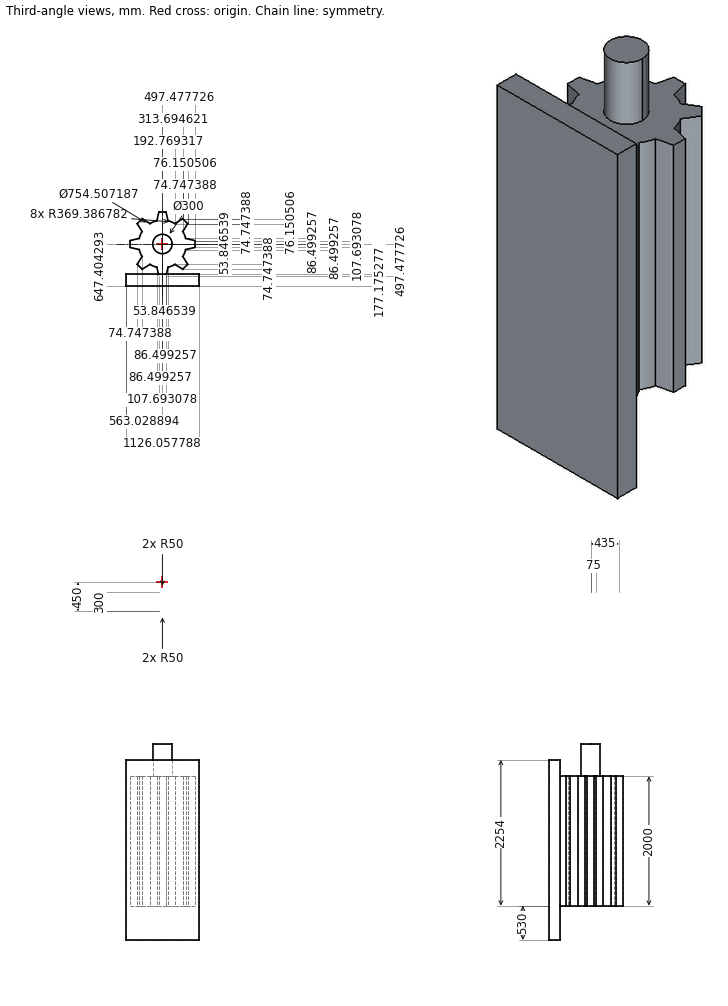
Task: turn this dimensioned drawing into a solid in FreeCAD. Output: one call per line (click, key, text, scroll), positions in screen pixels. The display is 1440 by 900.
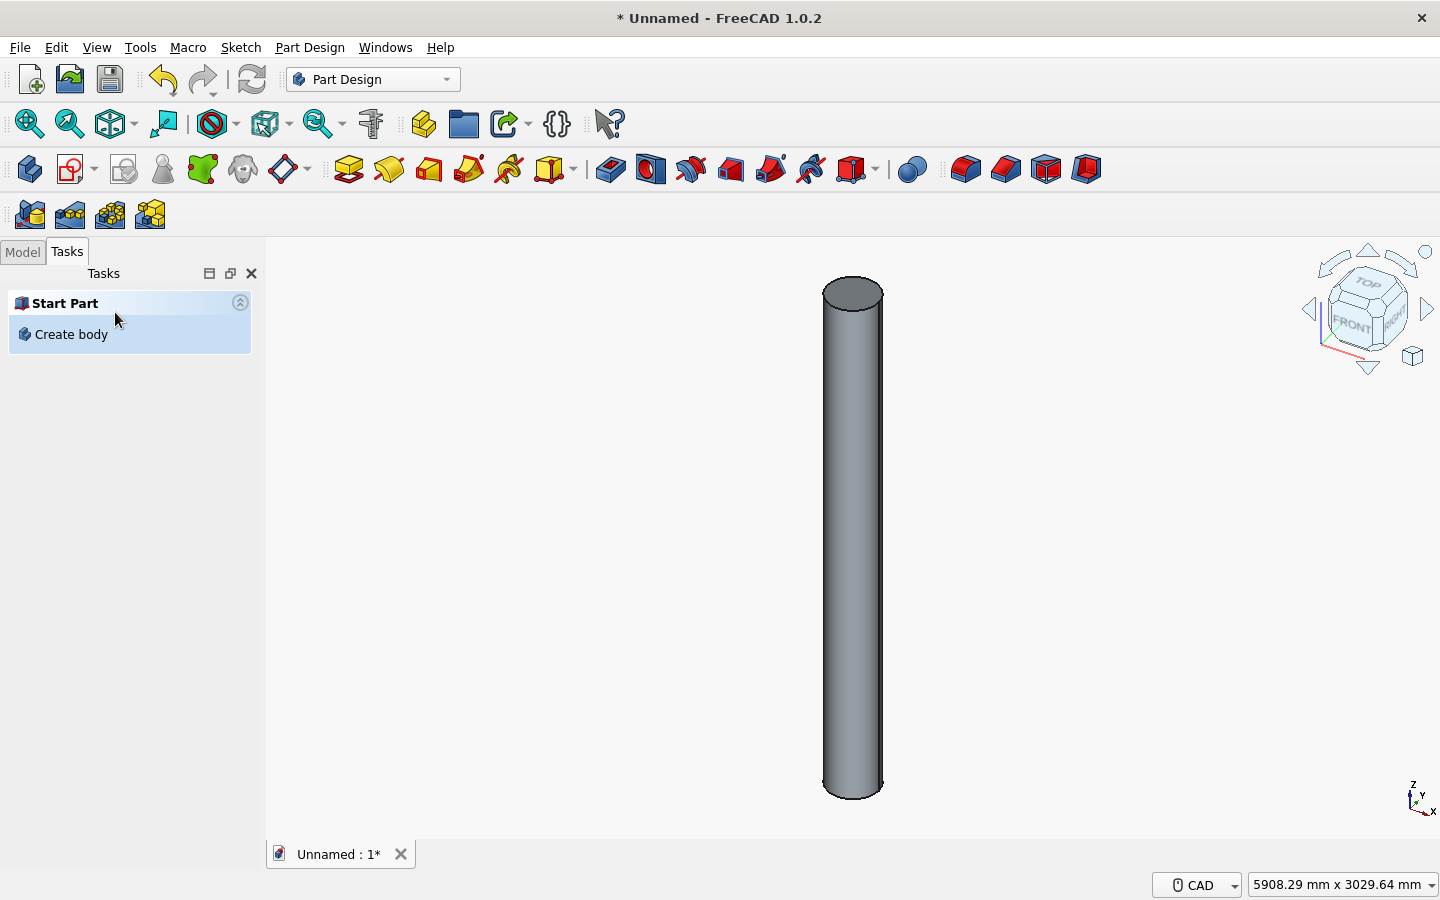
key(5)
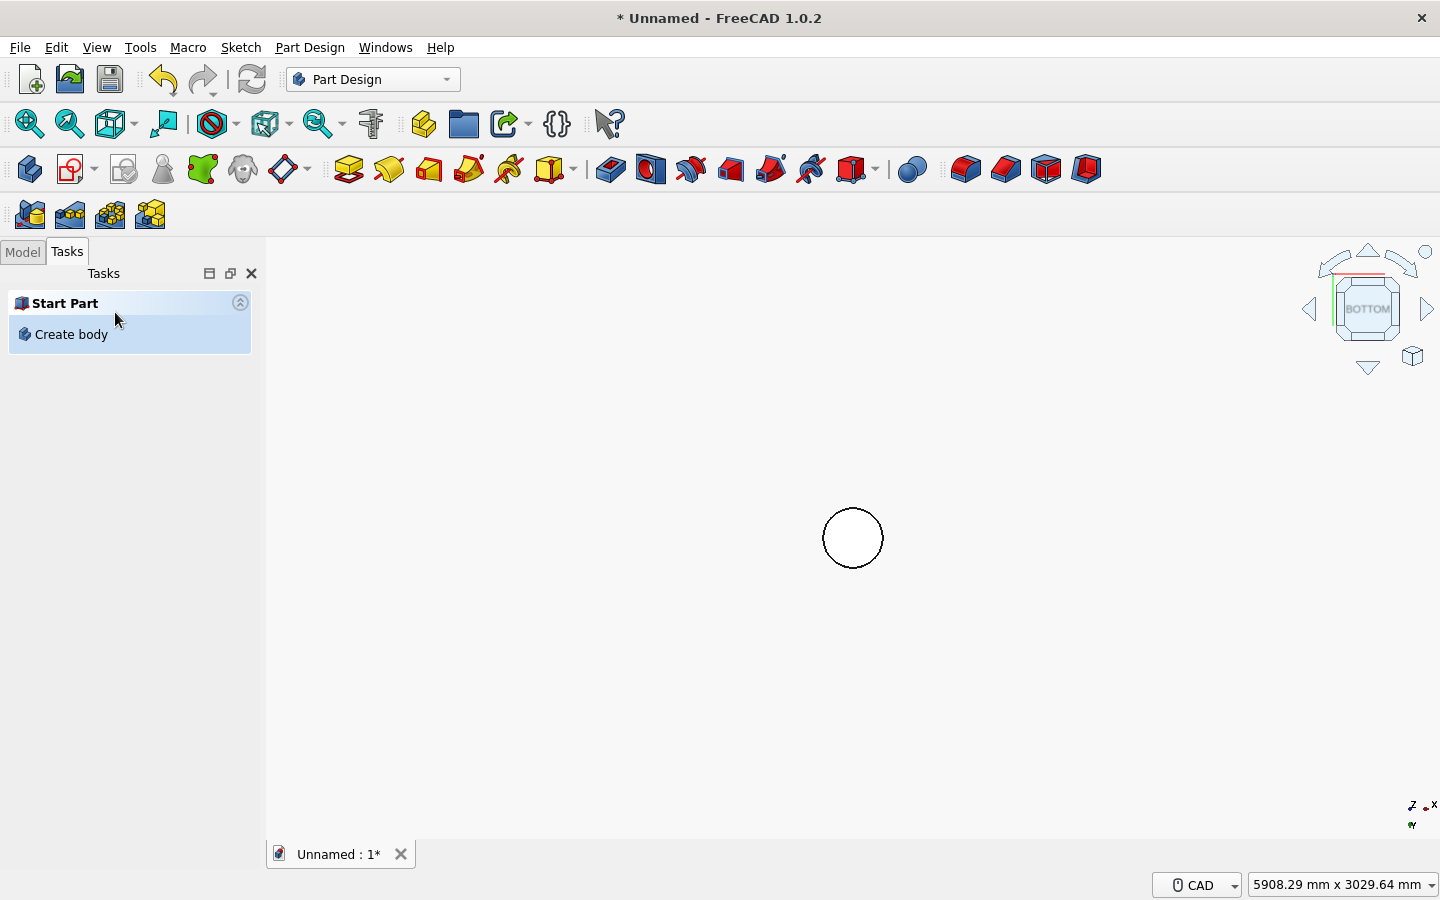
click(30, 124)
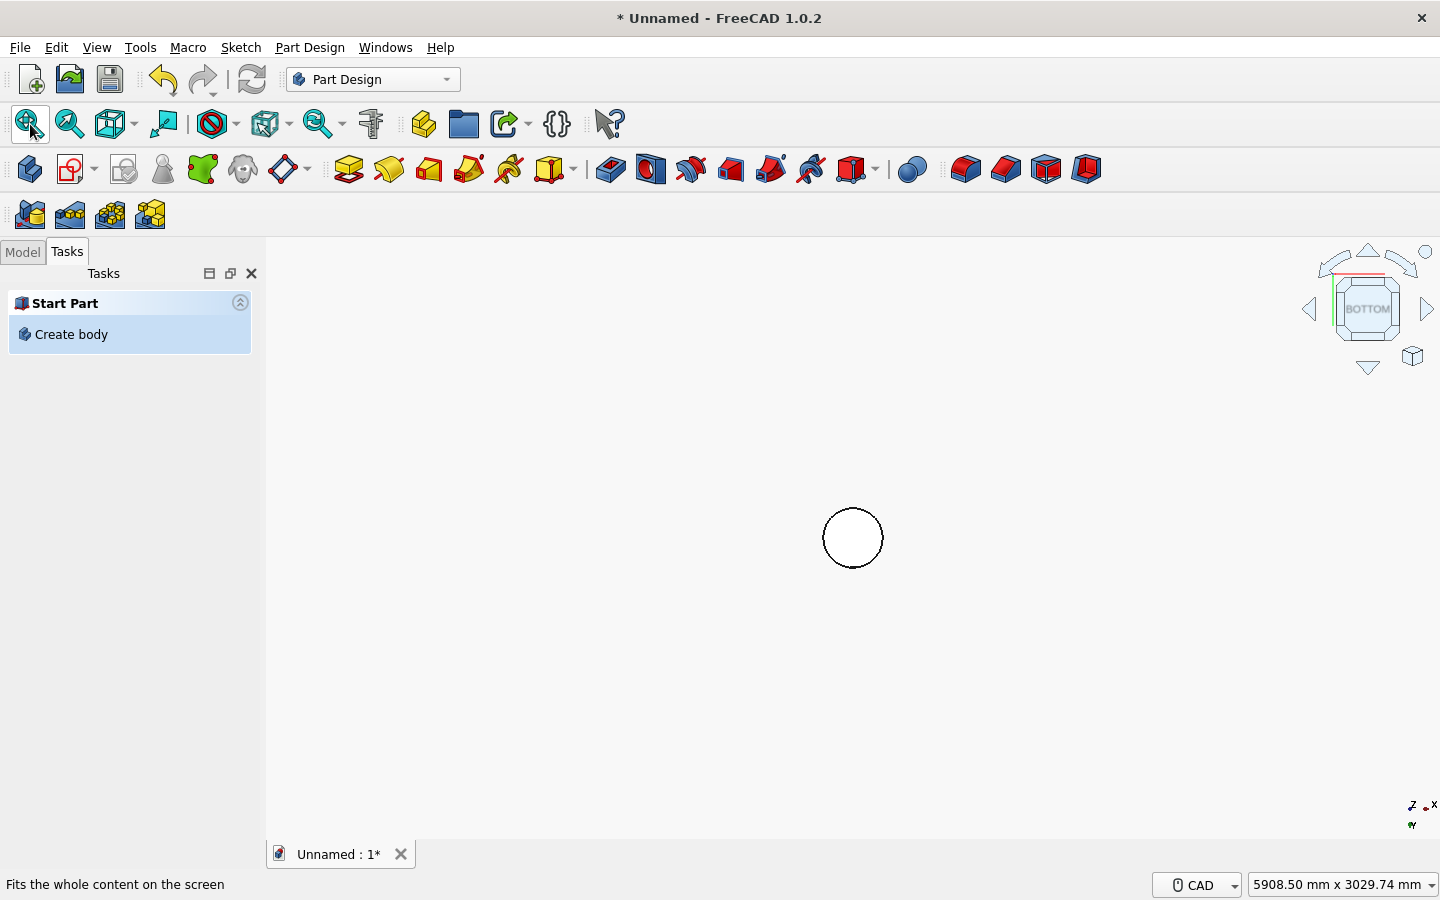
click(853, 537)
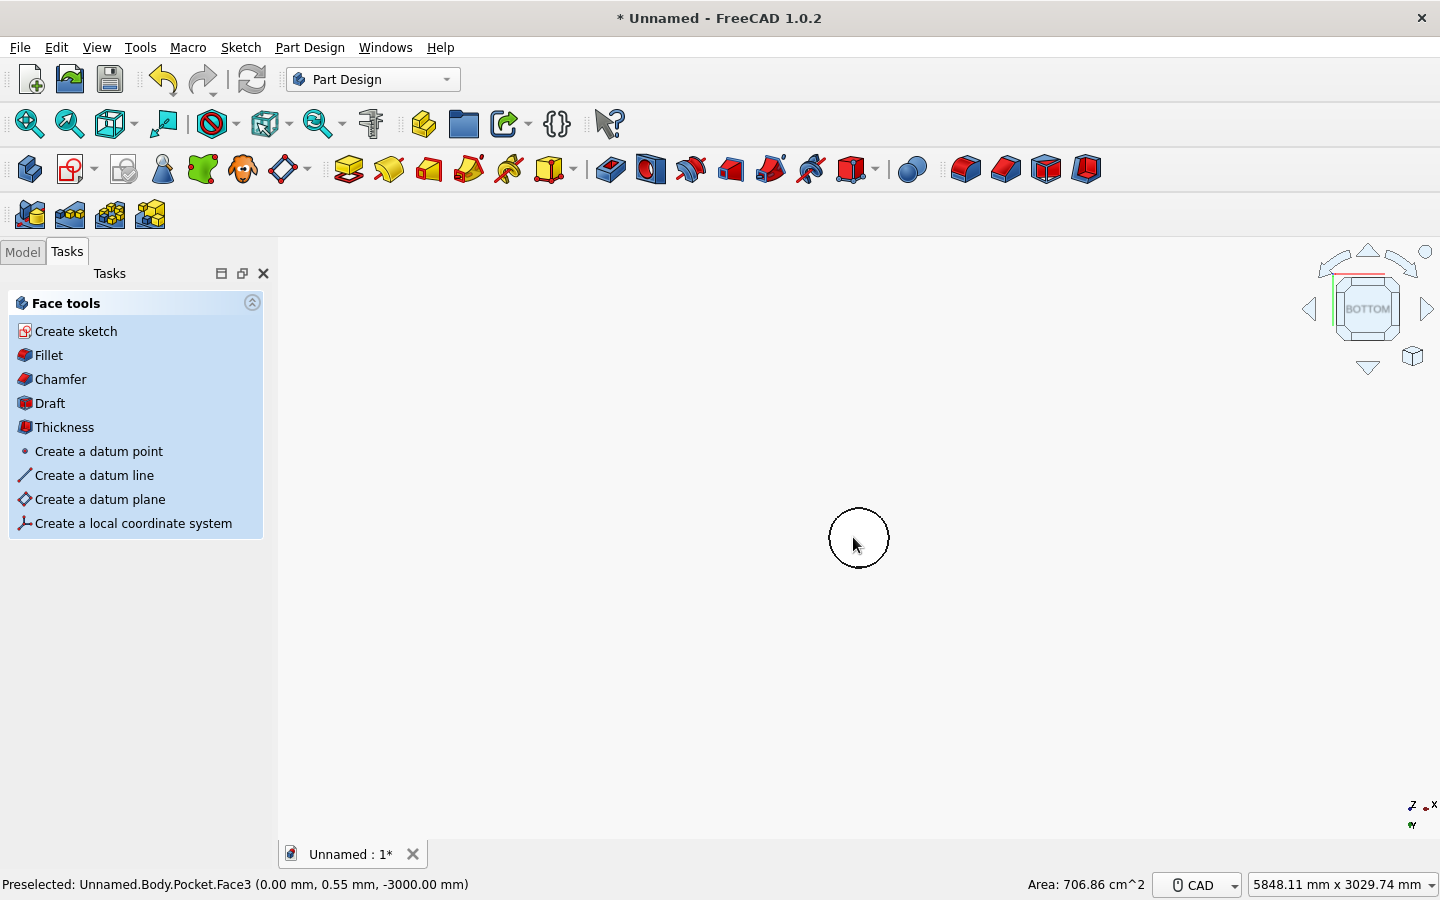
click(70, 170)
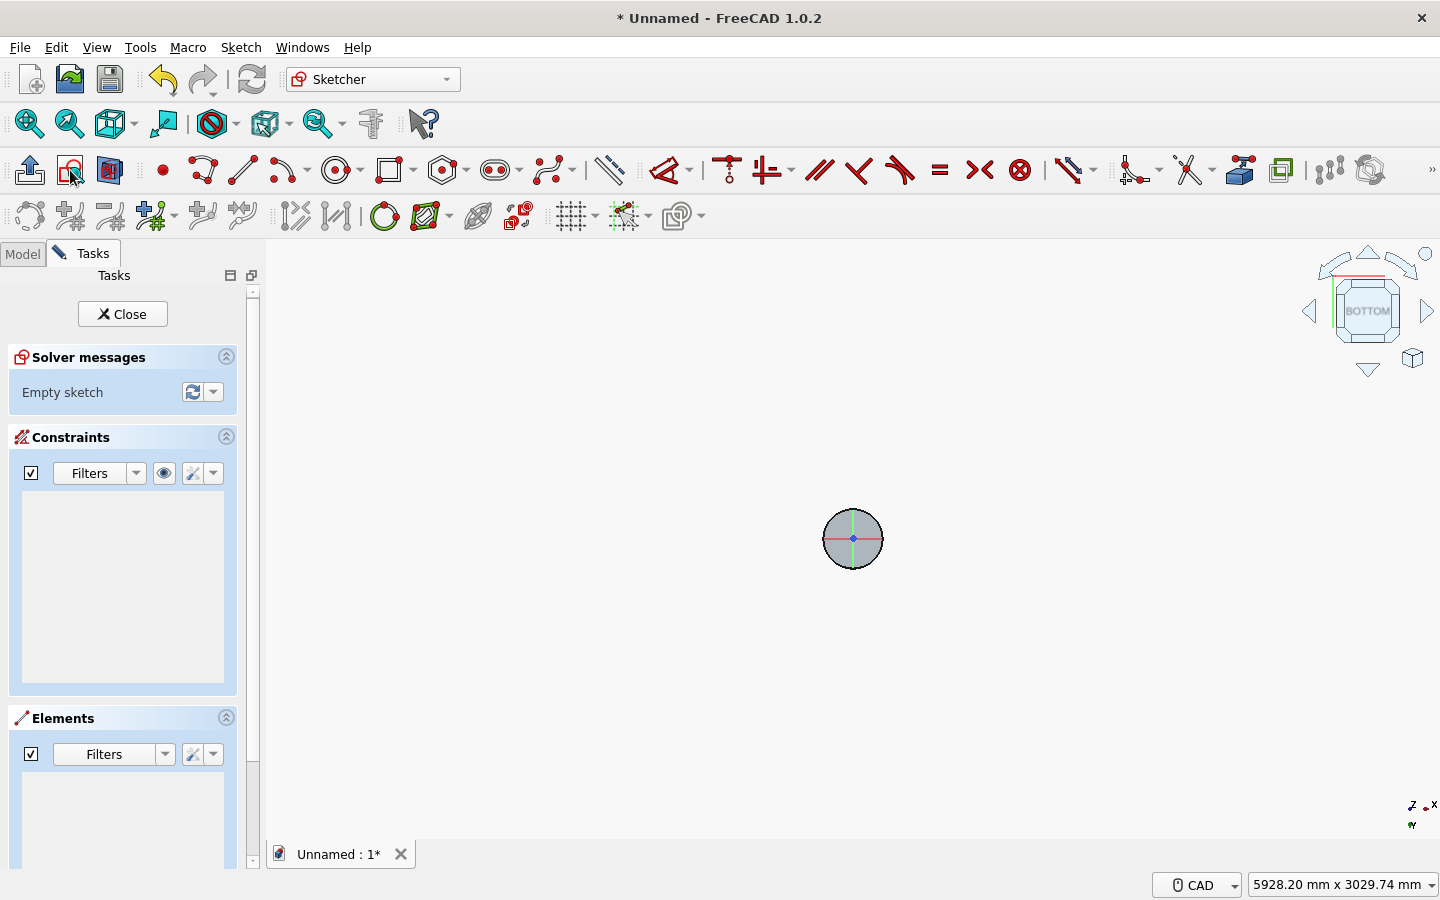
scroll(936, 539, up, 3)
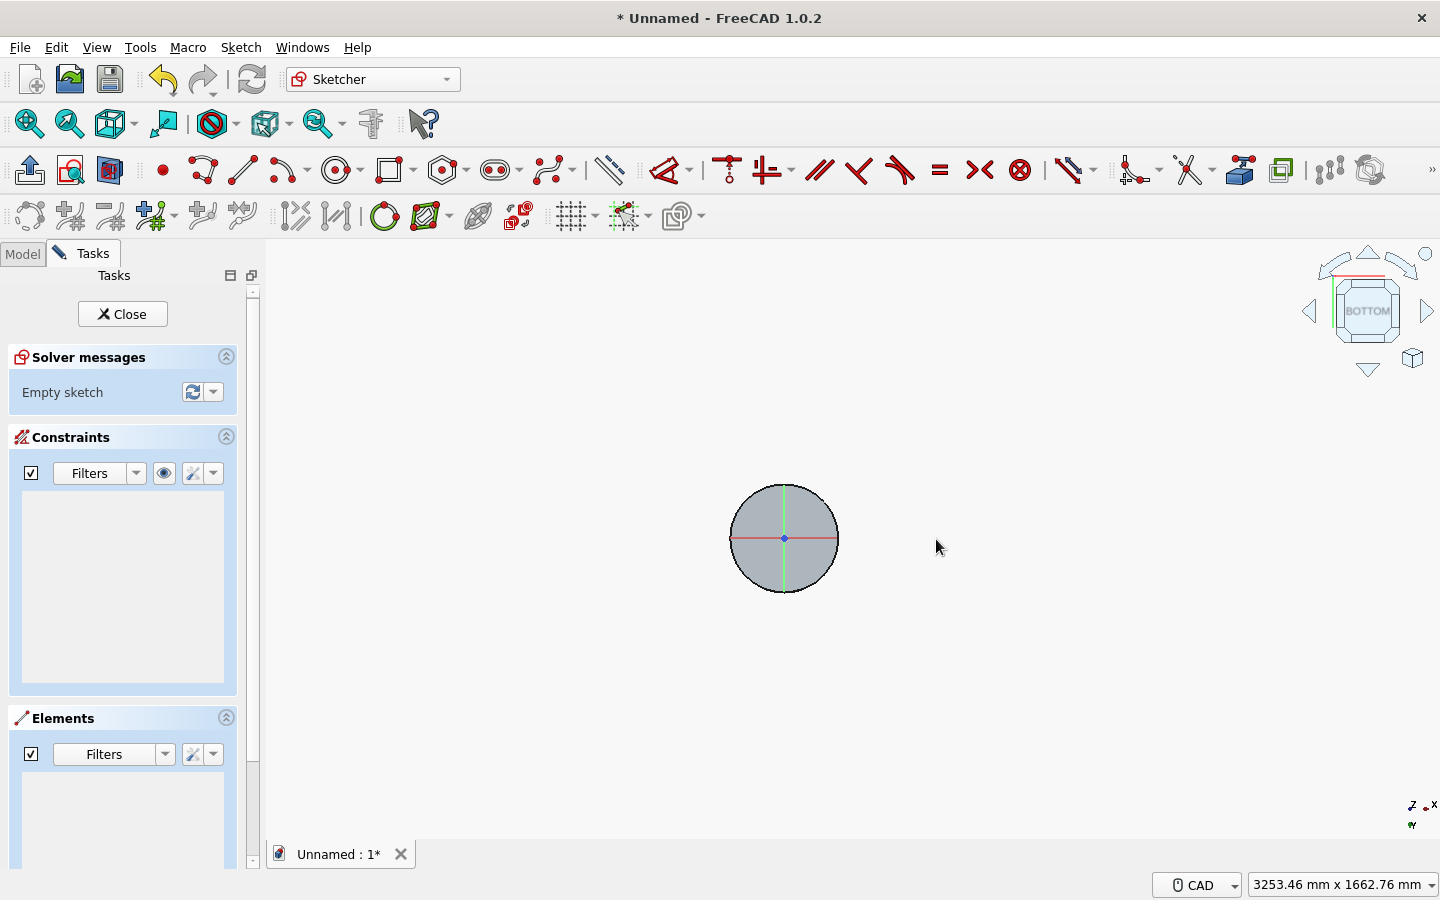
click(204, 170)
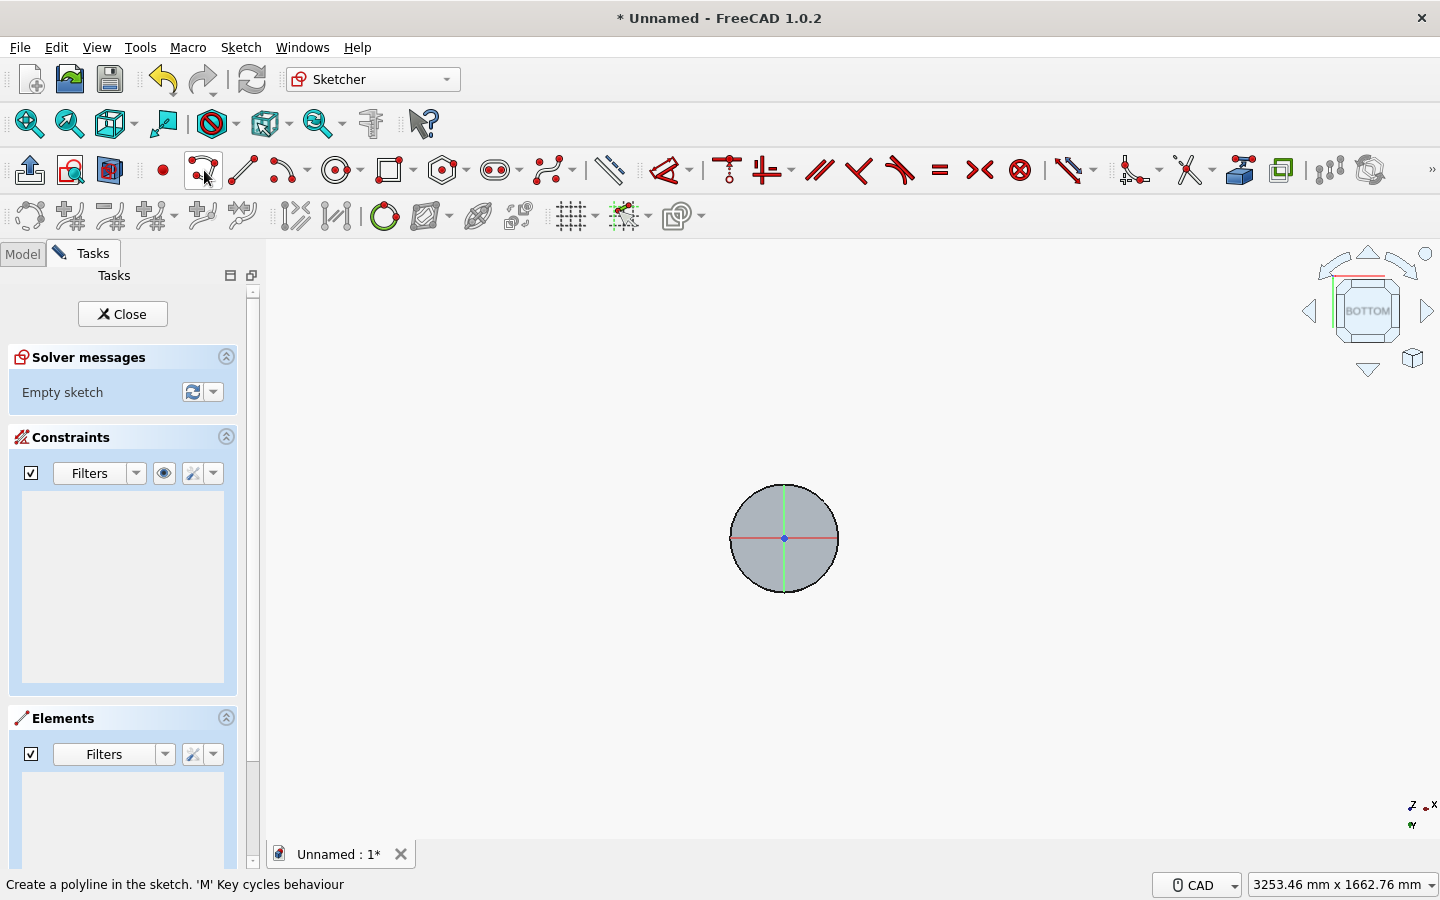
click(854, 652)
click(897, 679)
click(925, 652)
click(898, 608)
right_click(898, 608)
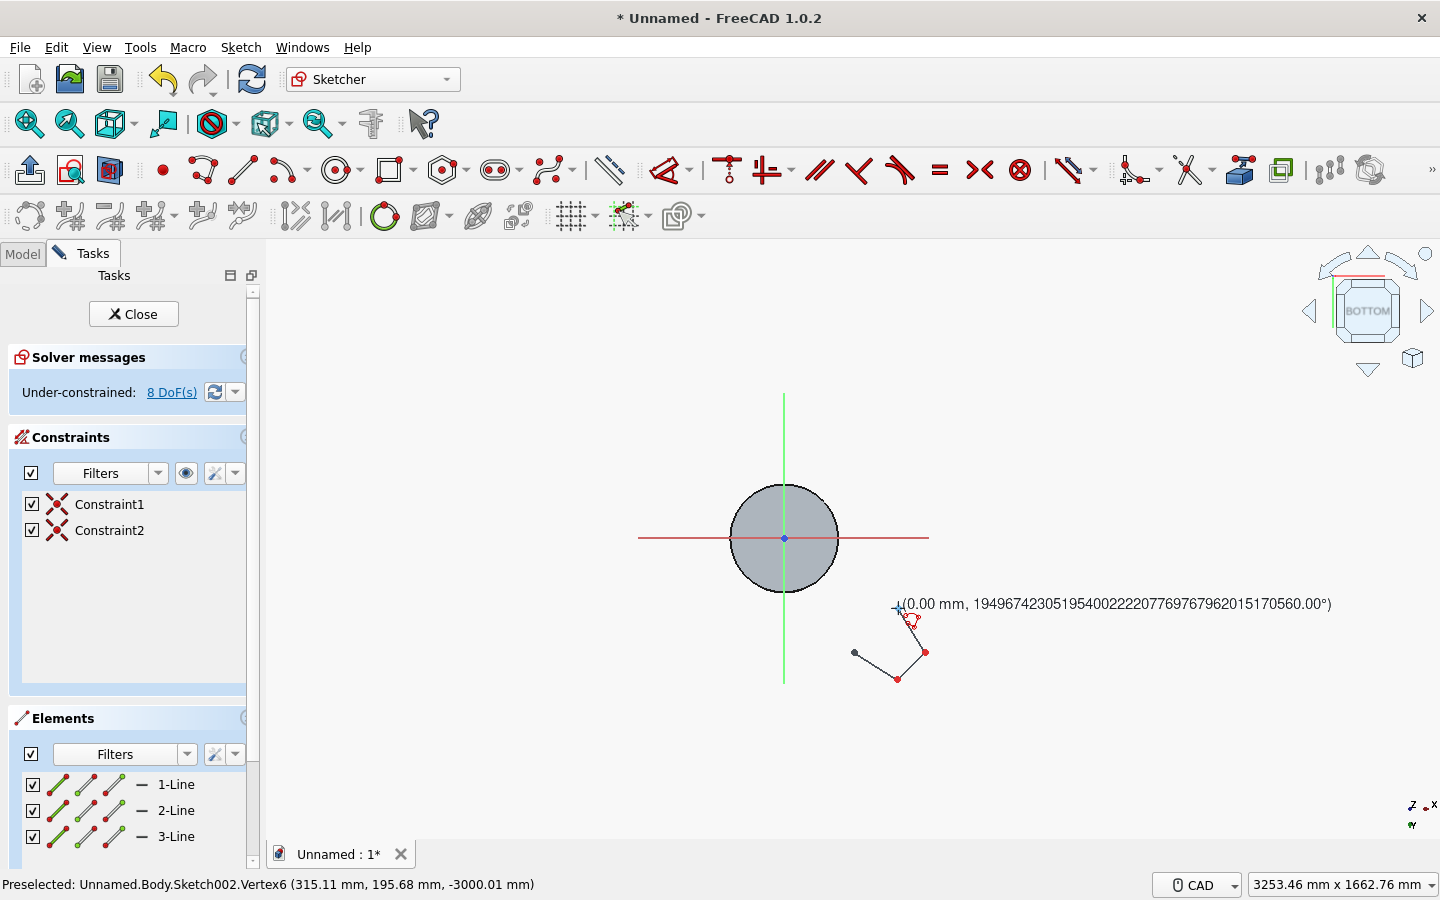
click(914, 570)
click(964, 558)
click(964, 519)
click(914, 507)
right_click(914, 507)